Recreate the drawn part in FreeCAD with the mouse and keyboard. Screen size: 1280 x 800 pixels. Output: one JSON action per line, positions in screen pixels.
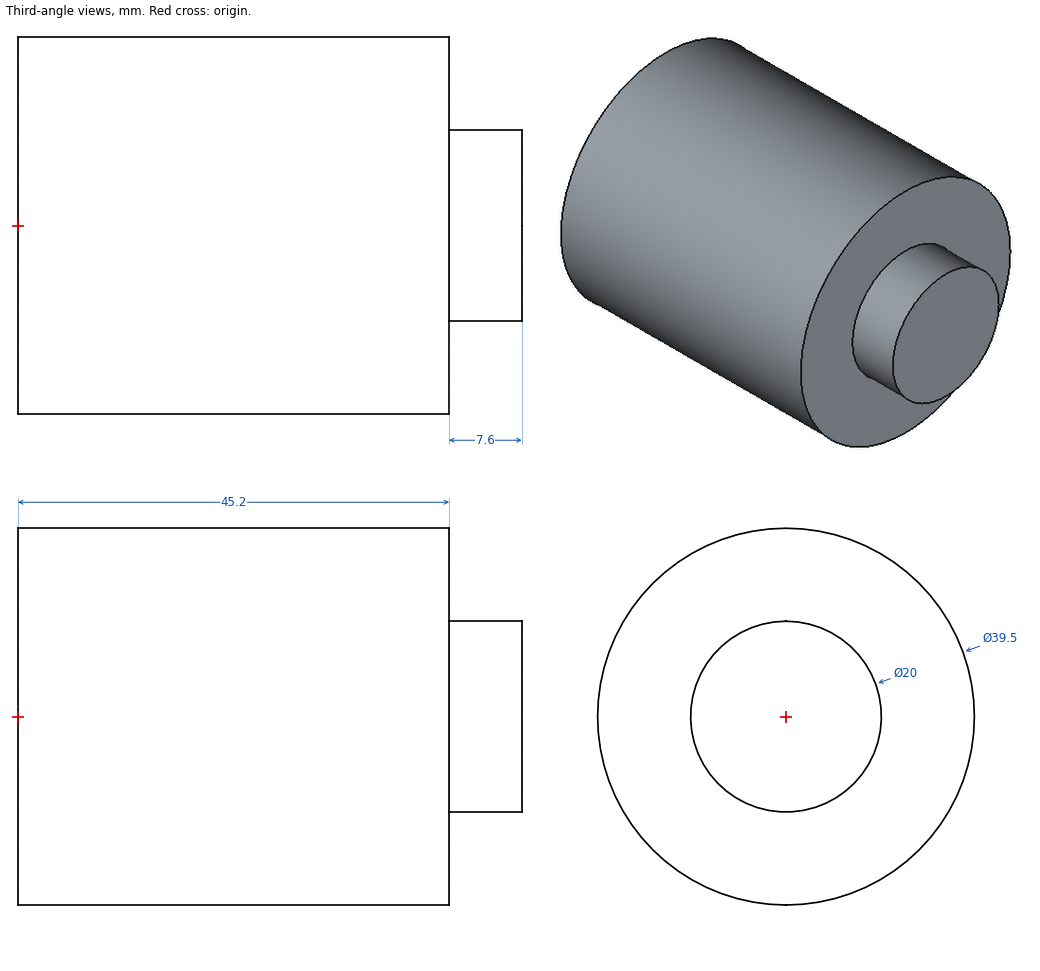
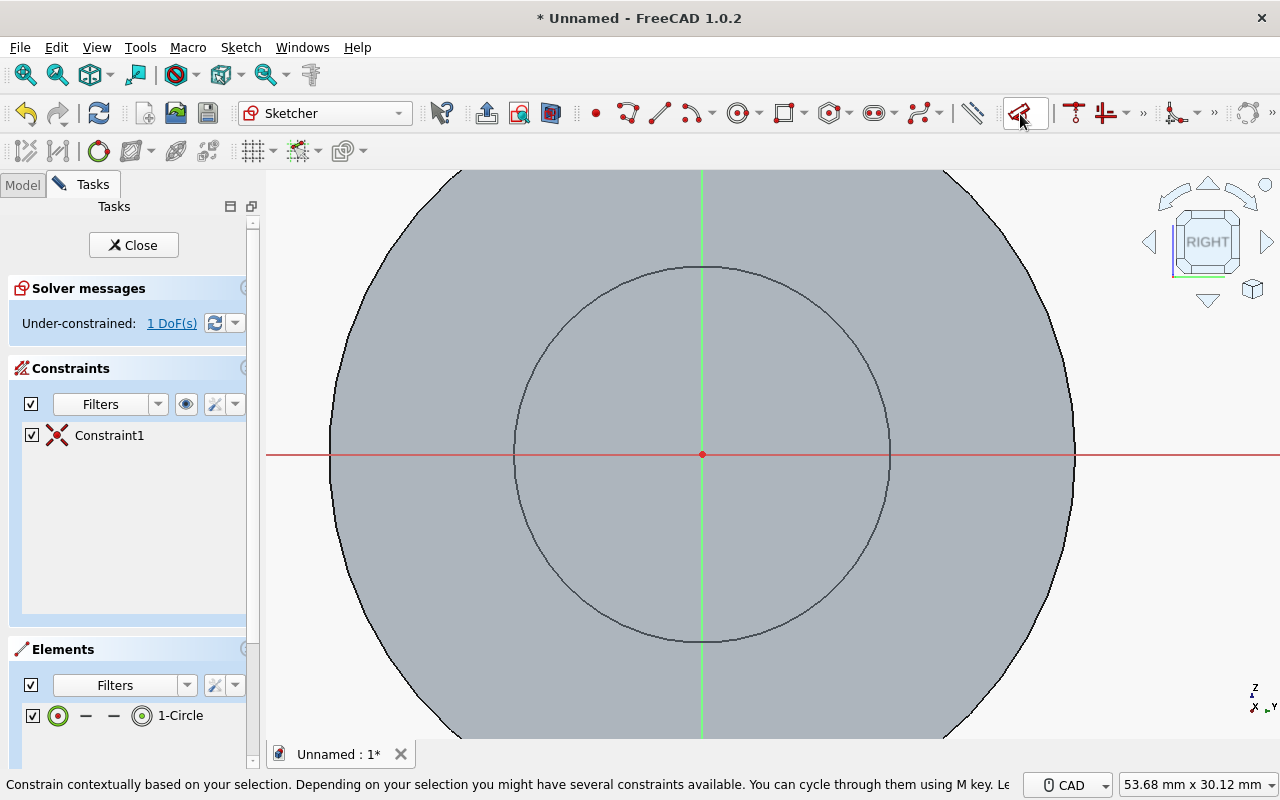
{"action": "left_click", "coordinate": [835, 321]}
{"action": "left_click", "coordinate": [858, 298]}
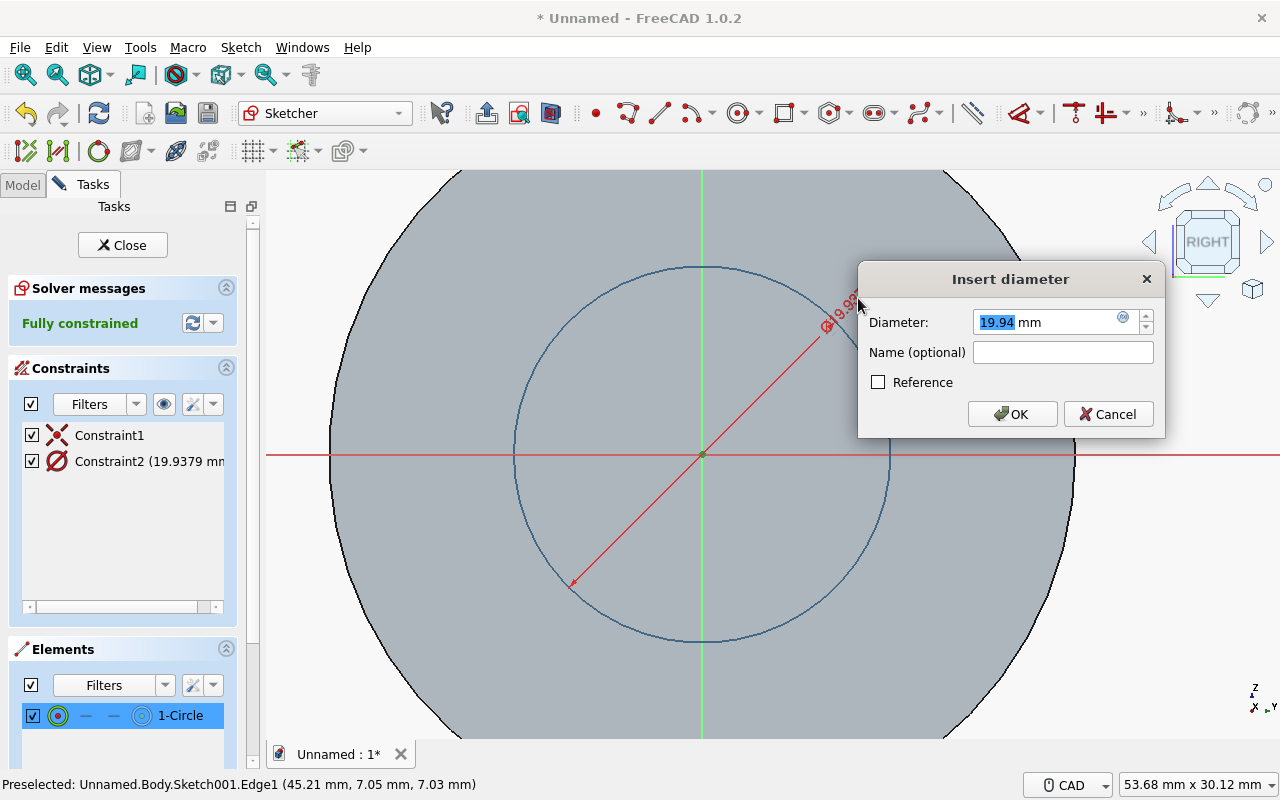
{"action": "type", "text": "20"}
{"action": "key", "text": "Return"}
{"action": "key", "text": "Escape"}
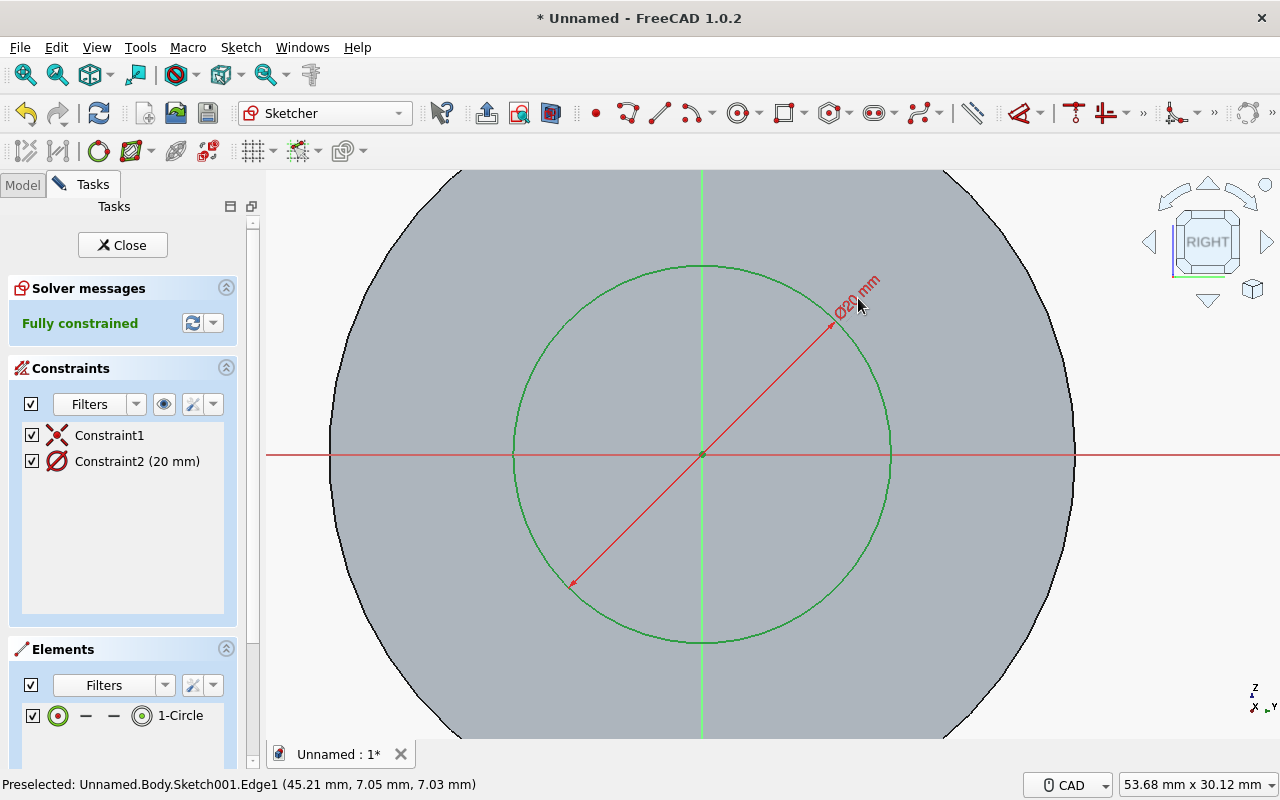
{"action": "left_click", "coordinate": [123, 245]}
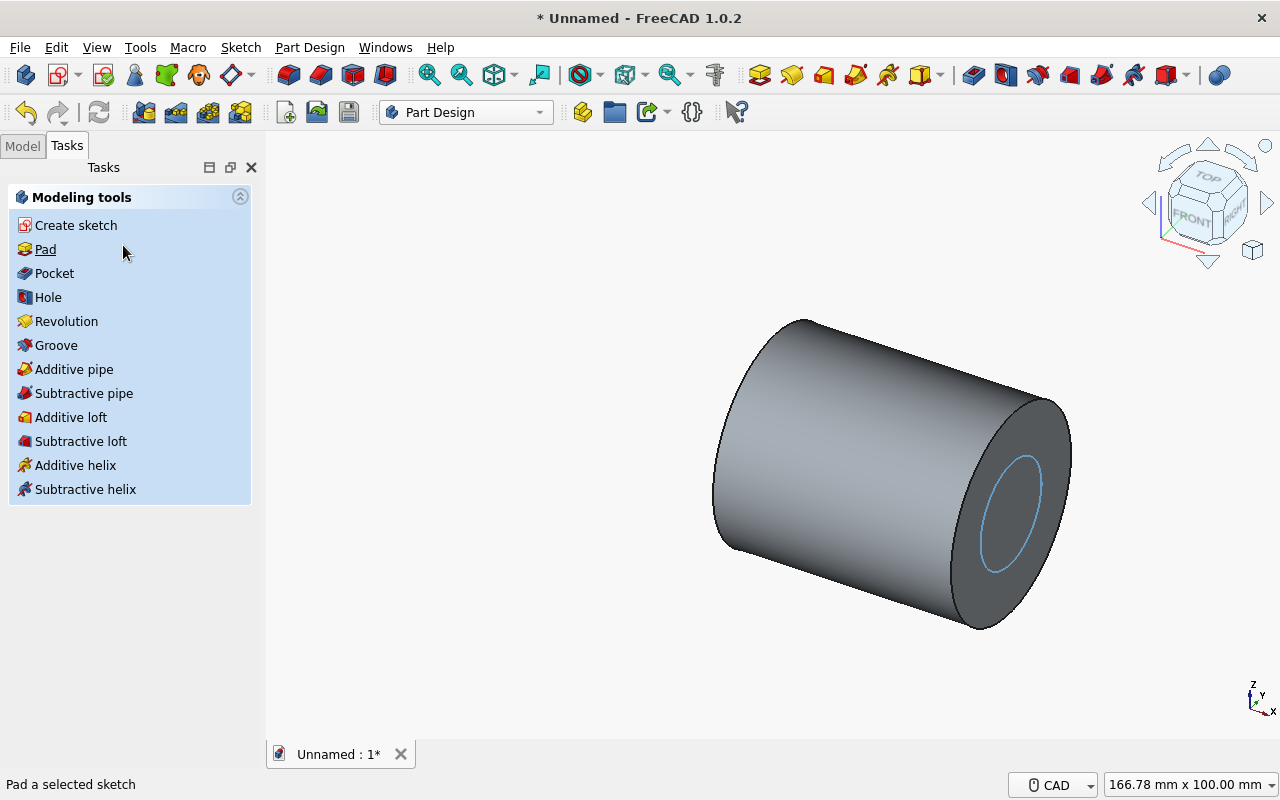
{"action": "left_click", "coordinate": [760, 76]}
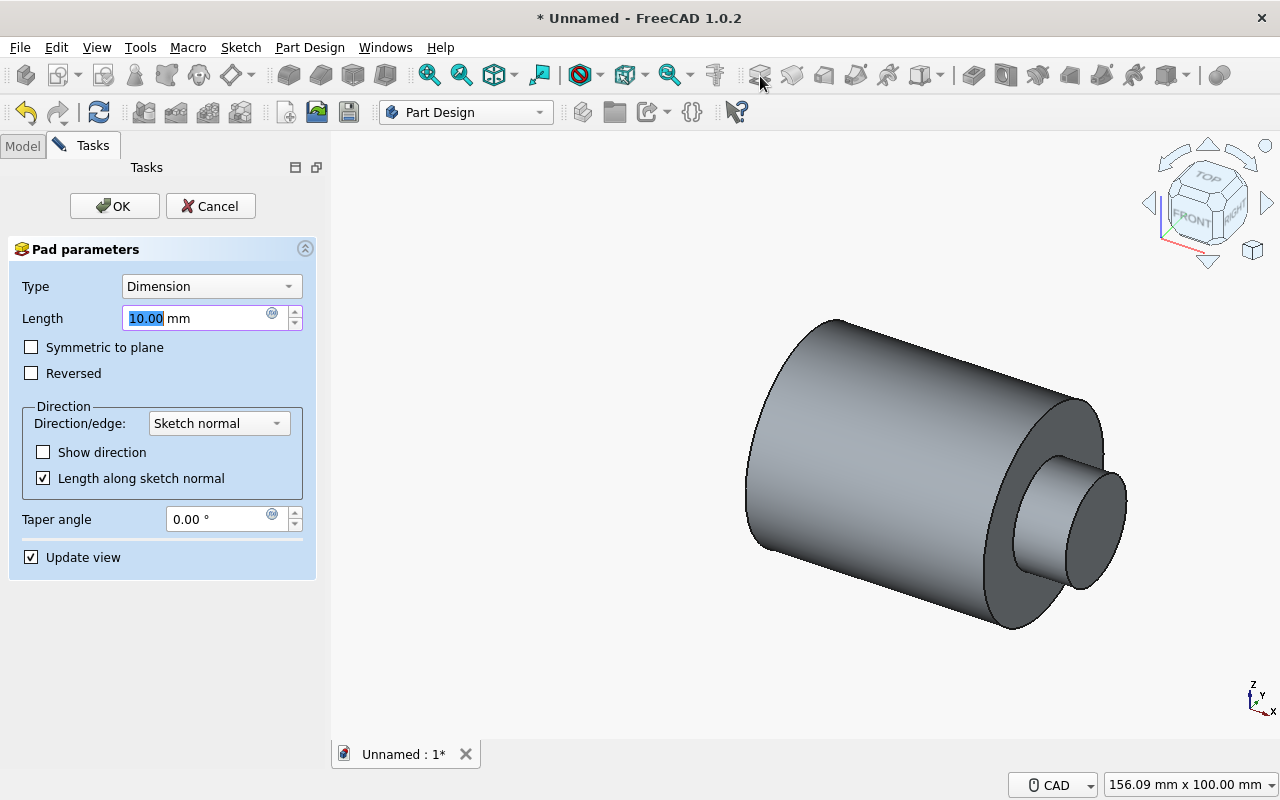
{"action": "type", "text": "7.6"}
{"action": "key", "text": "Tab"}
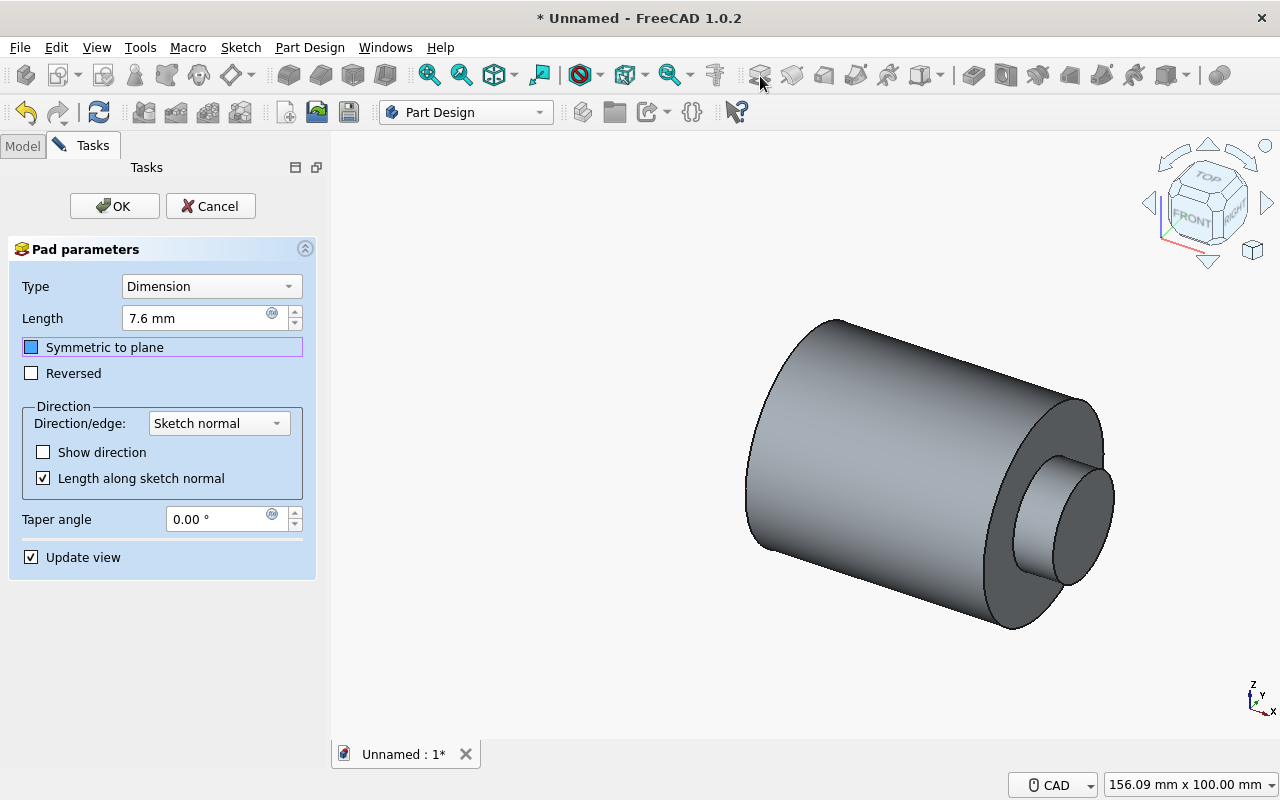
{"action": "left_click", "coordinate": [115, 206]}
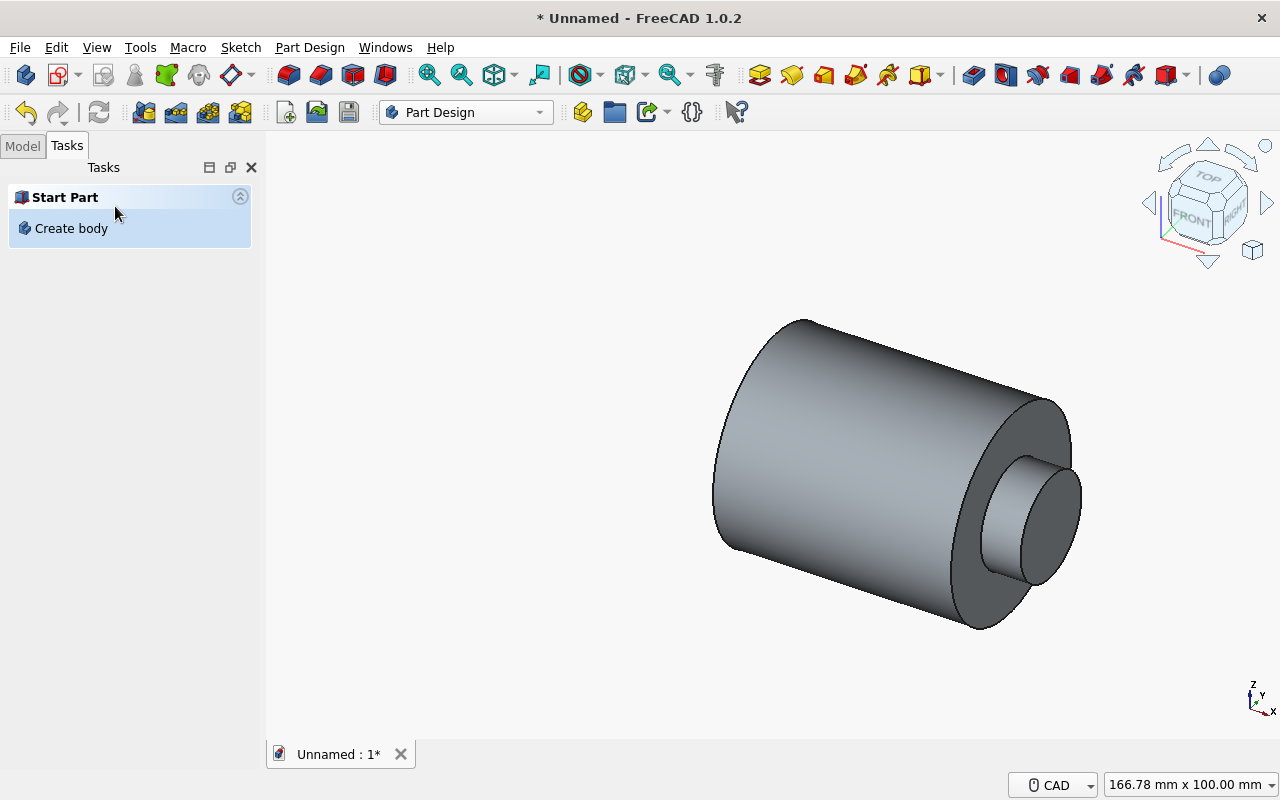
{"action": "key", "text": "0"}